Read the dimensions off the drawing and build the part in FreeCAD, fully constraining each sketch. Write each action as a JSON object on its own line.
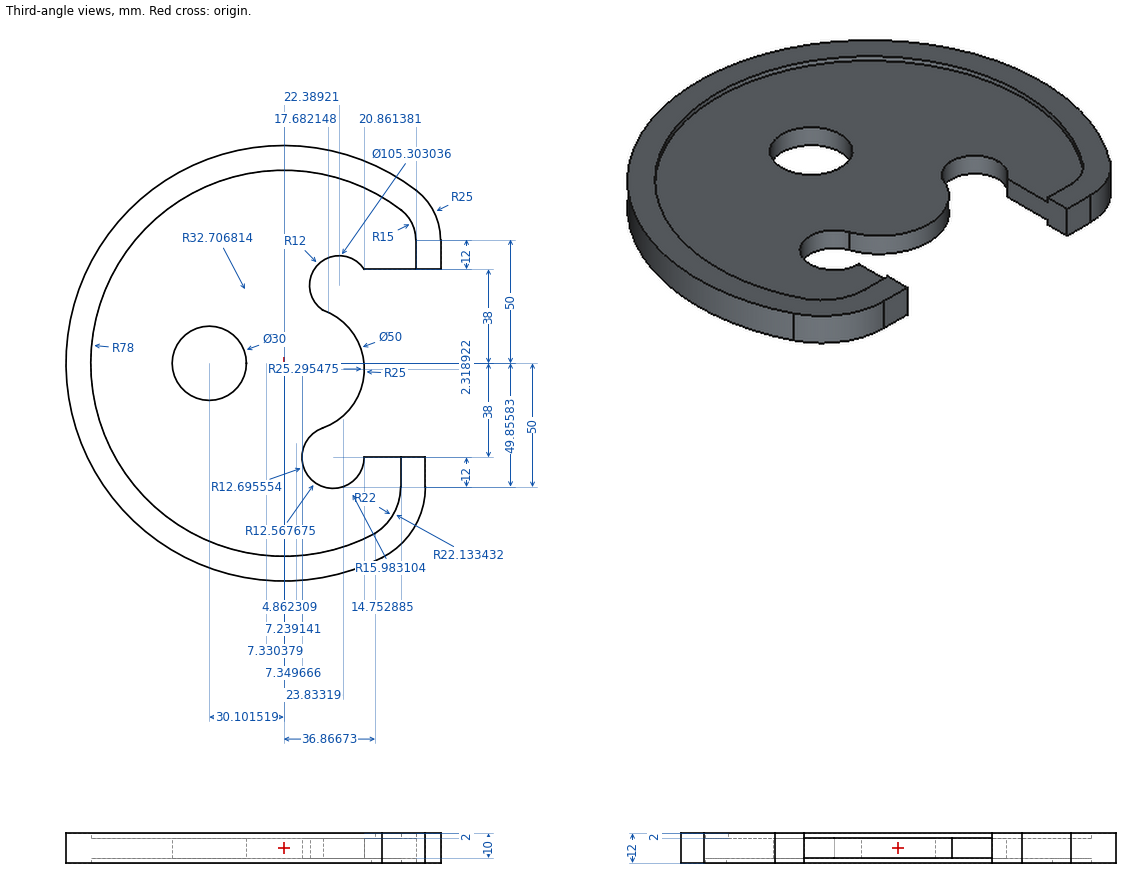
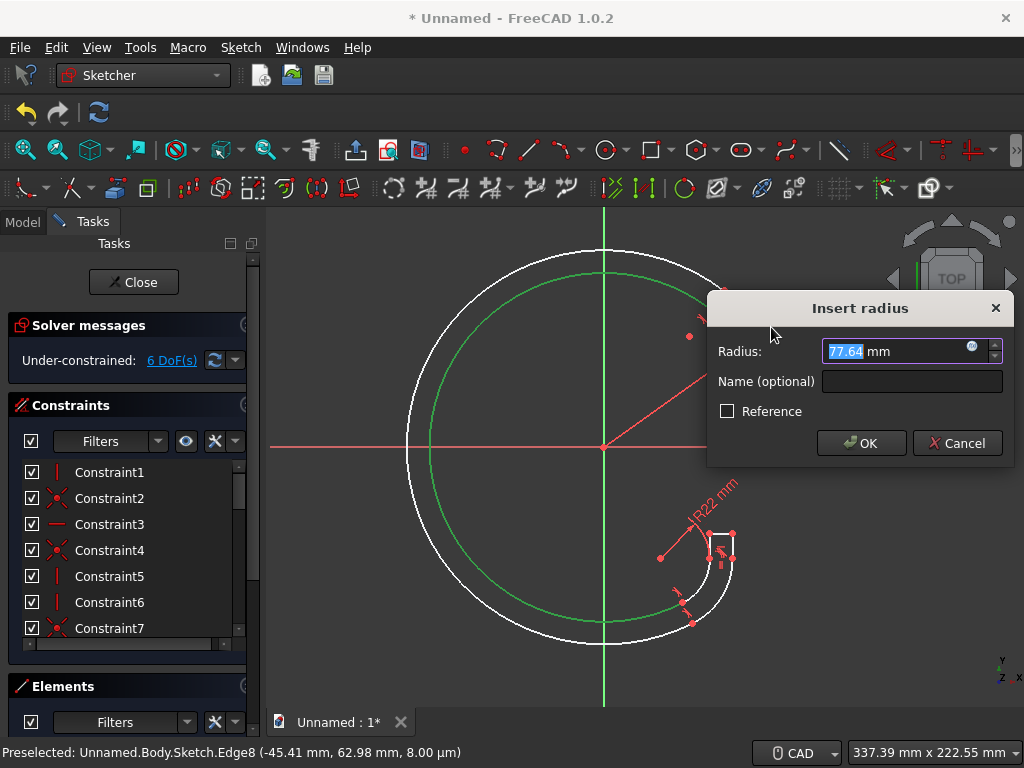
{"action": "type", "text": "78"}
{"action": "key", "text": "Return"}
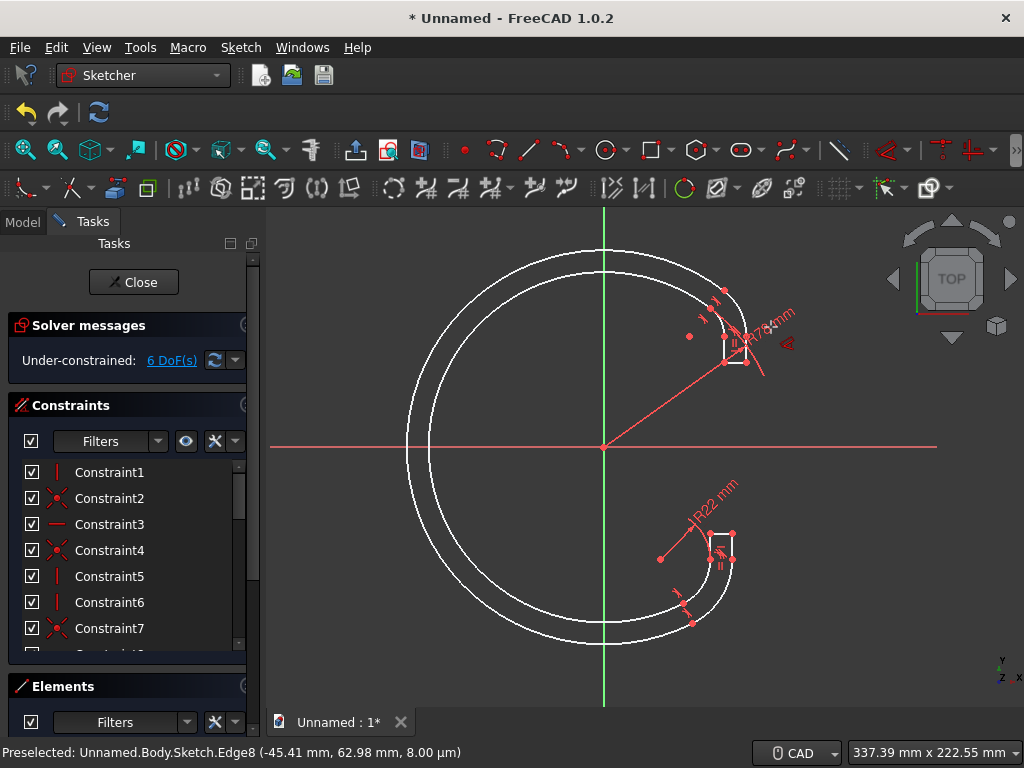
{"action": "scroll", "coordinate": [723, 327], "scroll_direction": "up", "scroll_amount": 2}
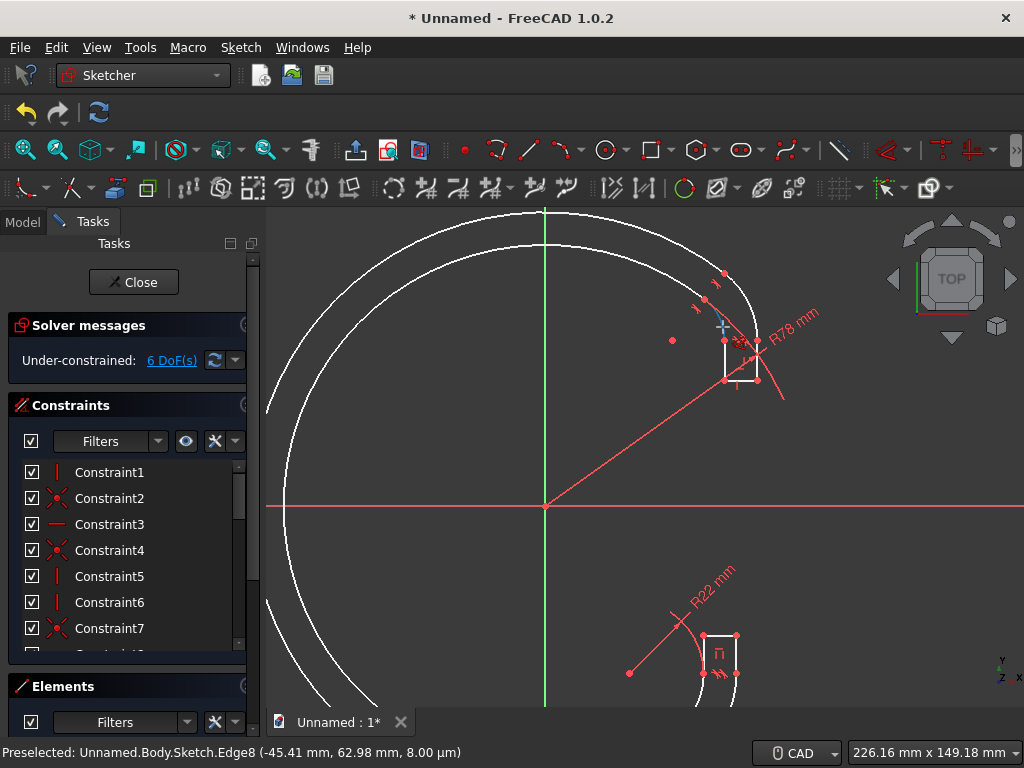
{"action": "left_click", "coordinate": [723, 326]}
{"action": "left_click", "coordinate": [736, 396]}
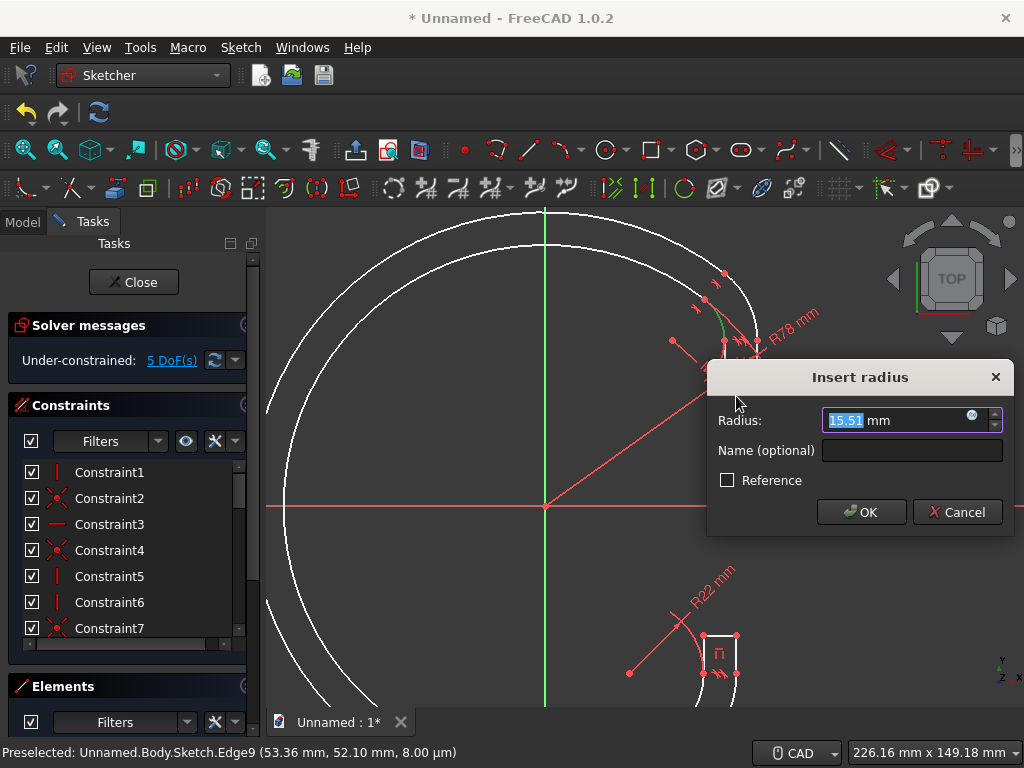
{"action": "type", "text": "15"}
{"action": "key", "text": "Return"}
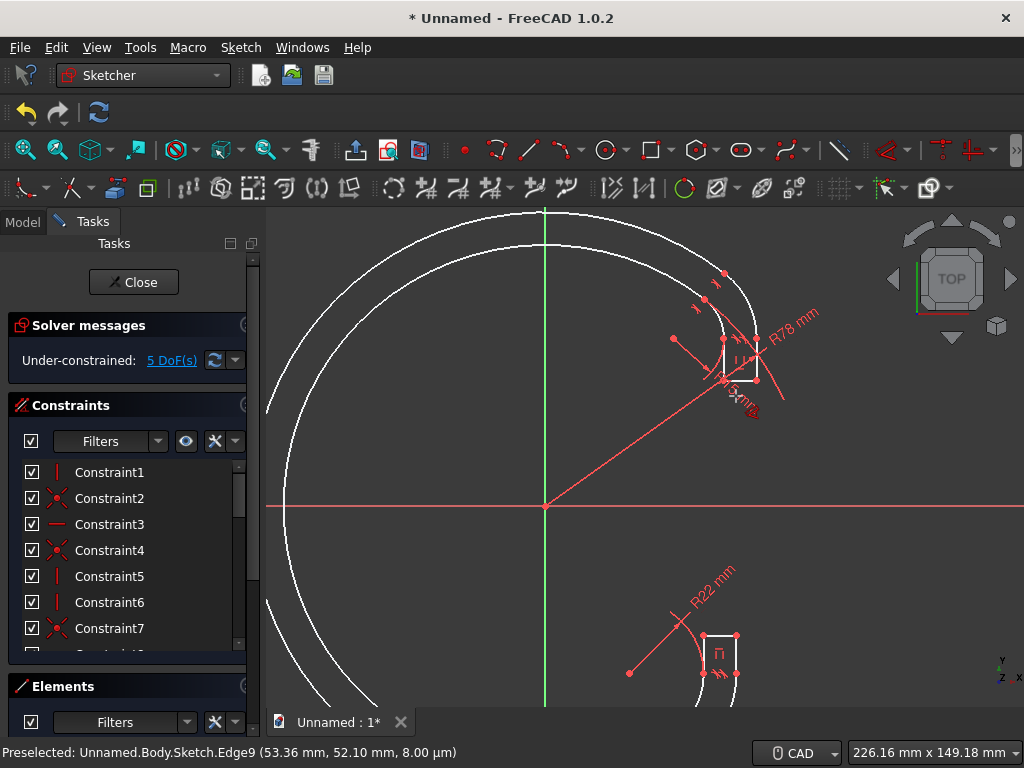
{"action": "left_click", "coordinate": [754, 316]}
{"action": "left_click", "coordinate": [786, 364]}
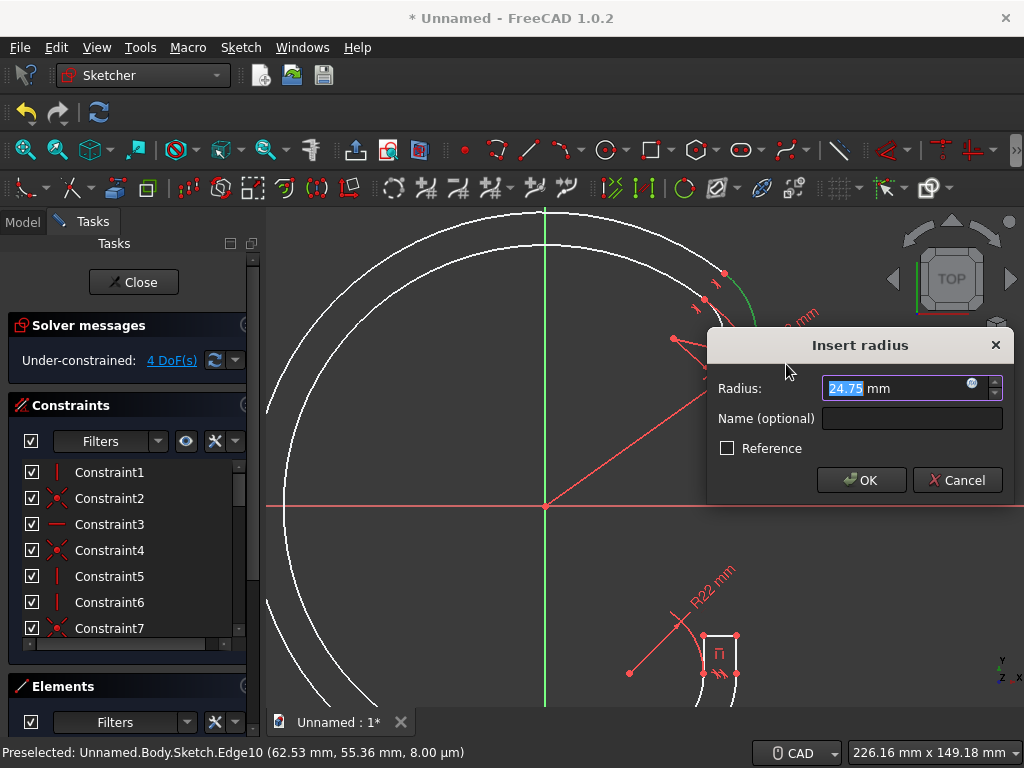
{"action": "type", "text": "25"}
{"action": "key", "text": "Return"}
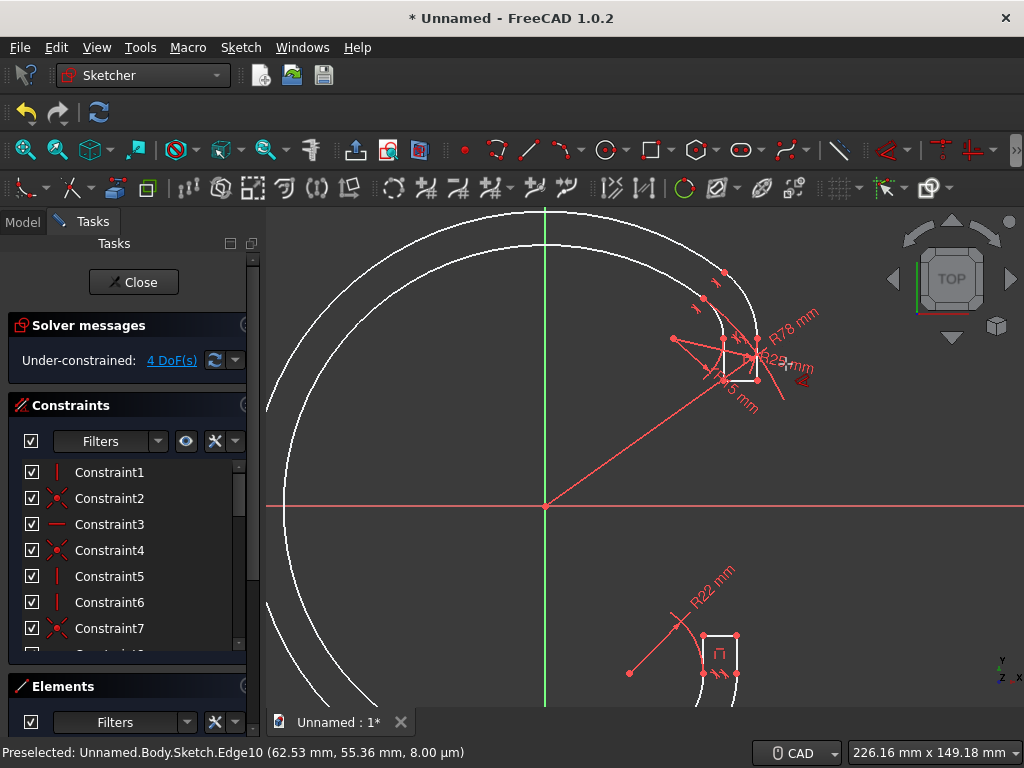
{"action": "left_click", "coordinate": [737, 662]}
{"action": "left_click", "coordinate": [771, 655]}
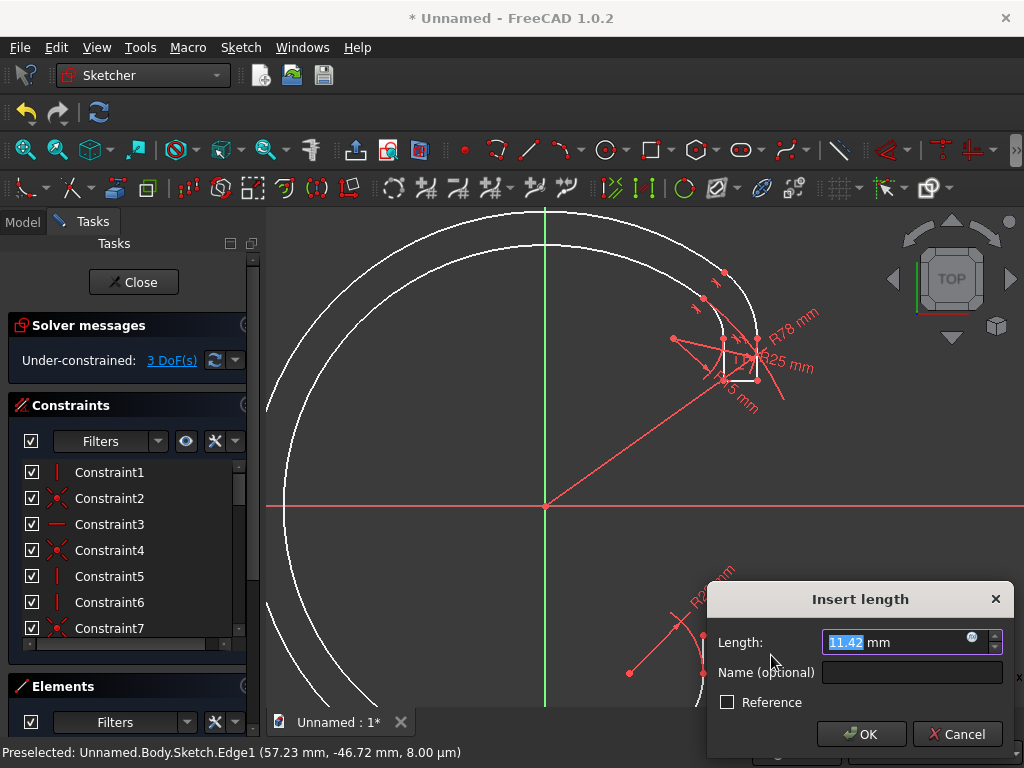
{"action": "type", "text": "12"}
{"action": "key", "text": "Return"}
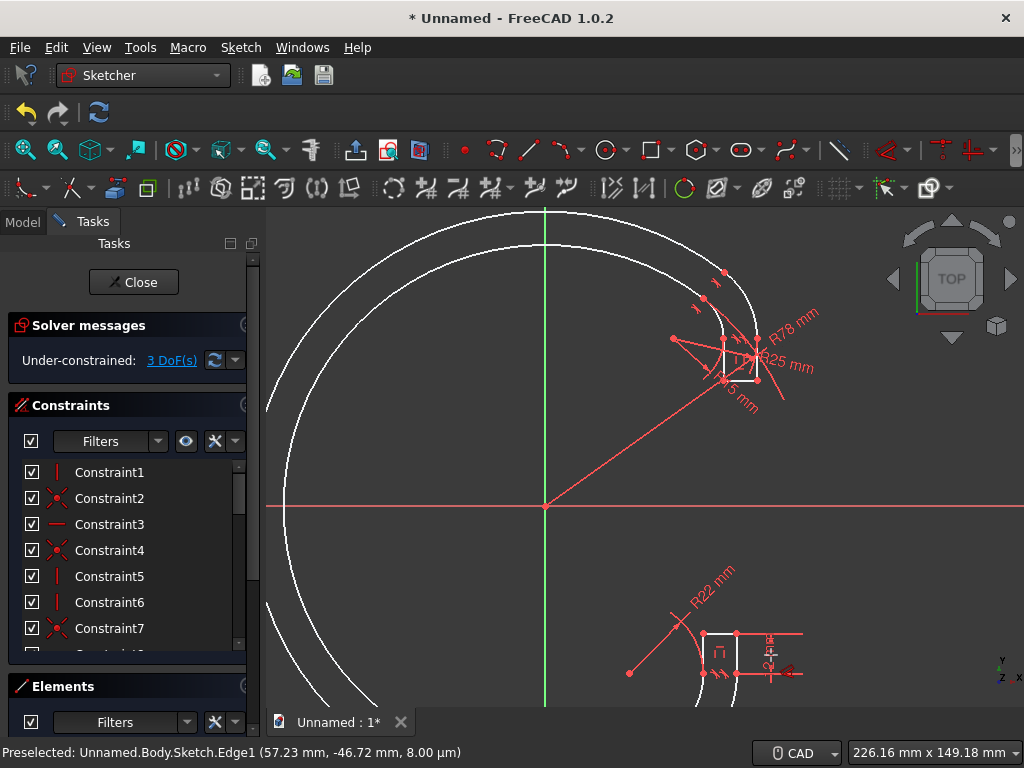
{"action": "left_click", "coordinate": [724, 351]}
{"action": "left_click", "coordinate": [690, 360]}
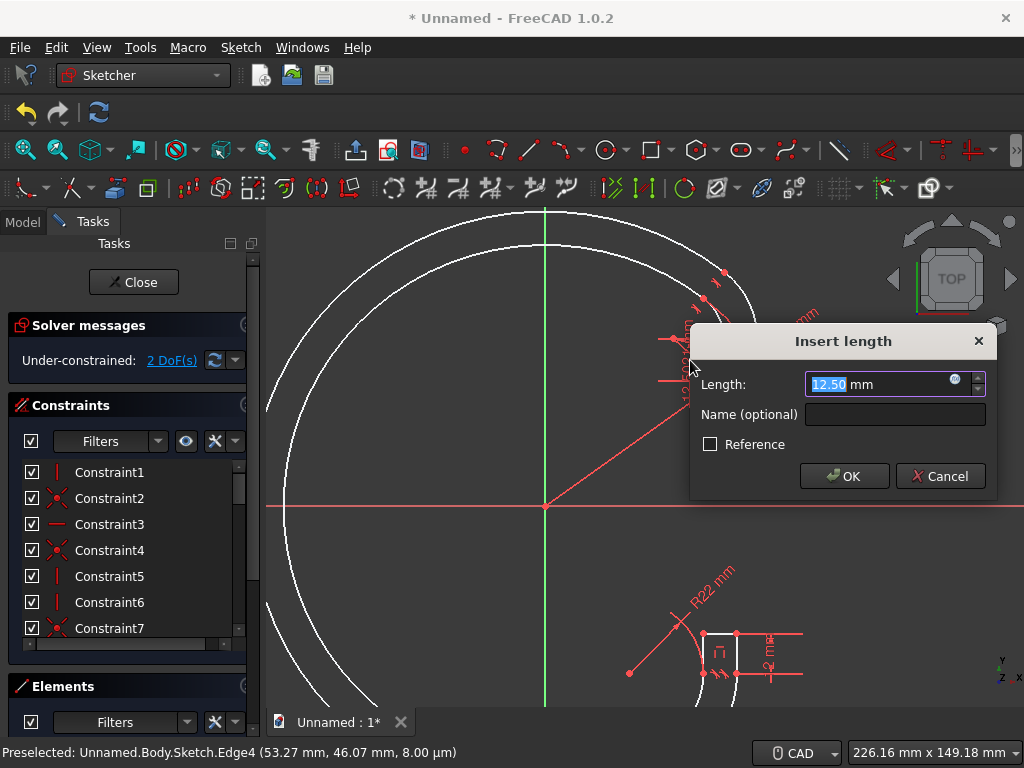
{"action": "type", "text": "12"}
{"action": "key", "text": "Return"}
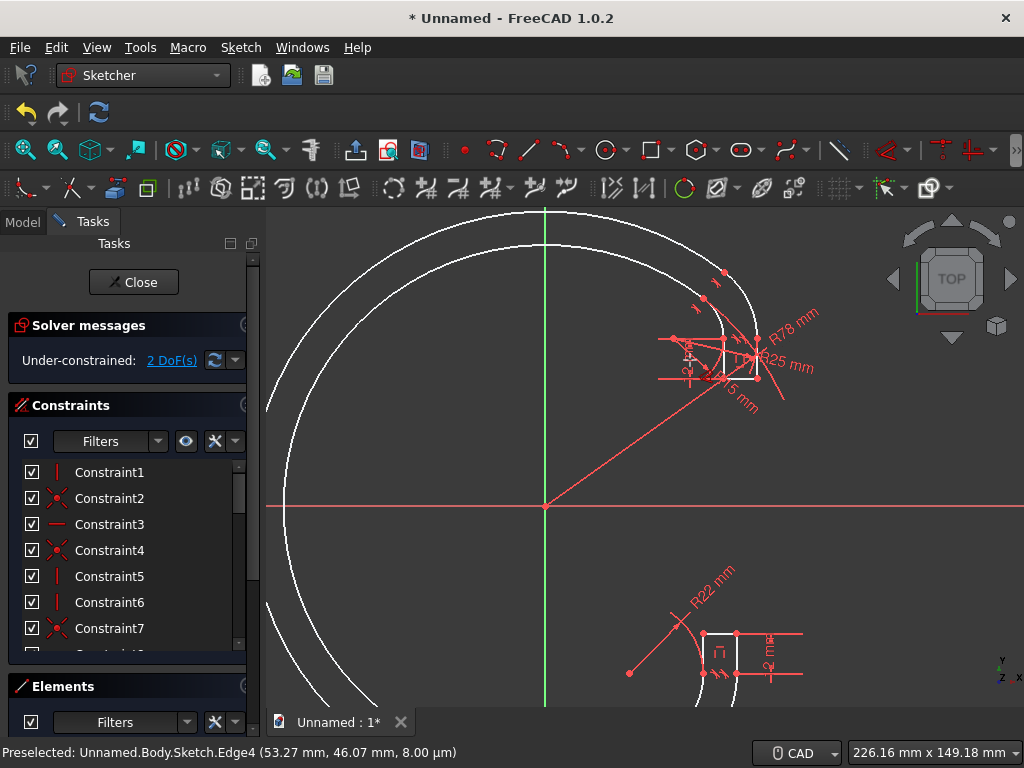
{"action": "left_click", "coordinate": [737, 674]}
{"action": "left_click", "coordinate": [771, 552]}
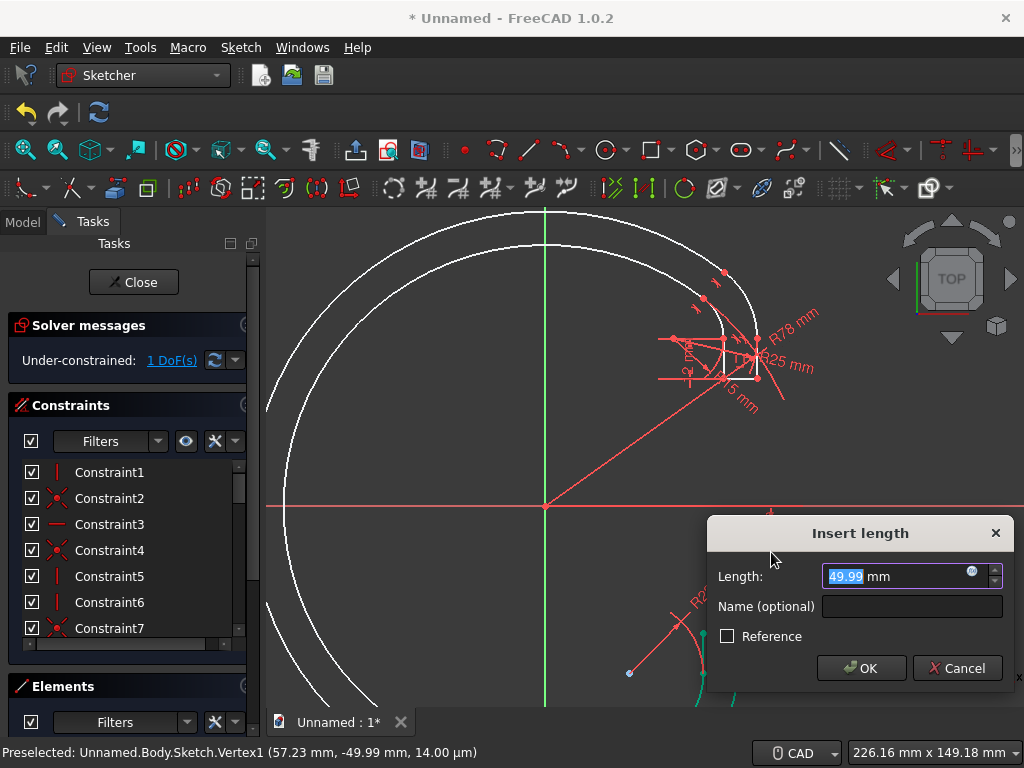
{"action": "type", "text": "50"}
{"action": "key", "text": "Return"}